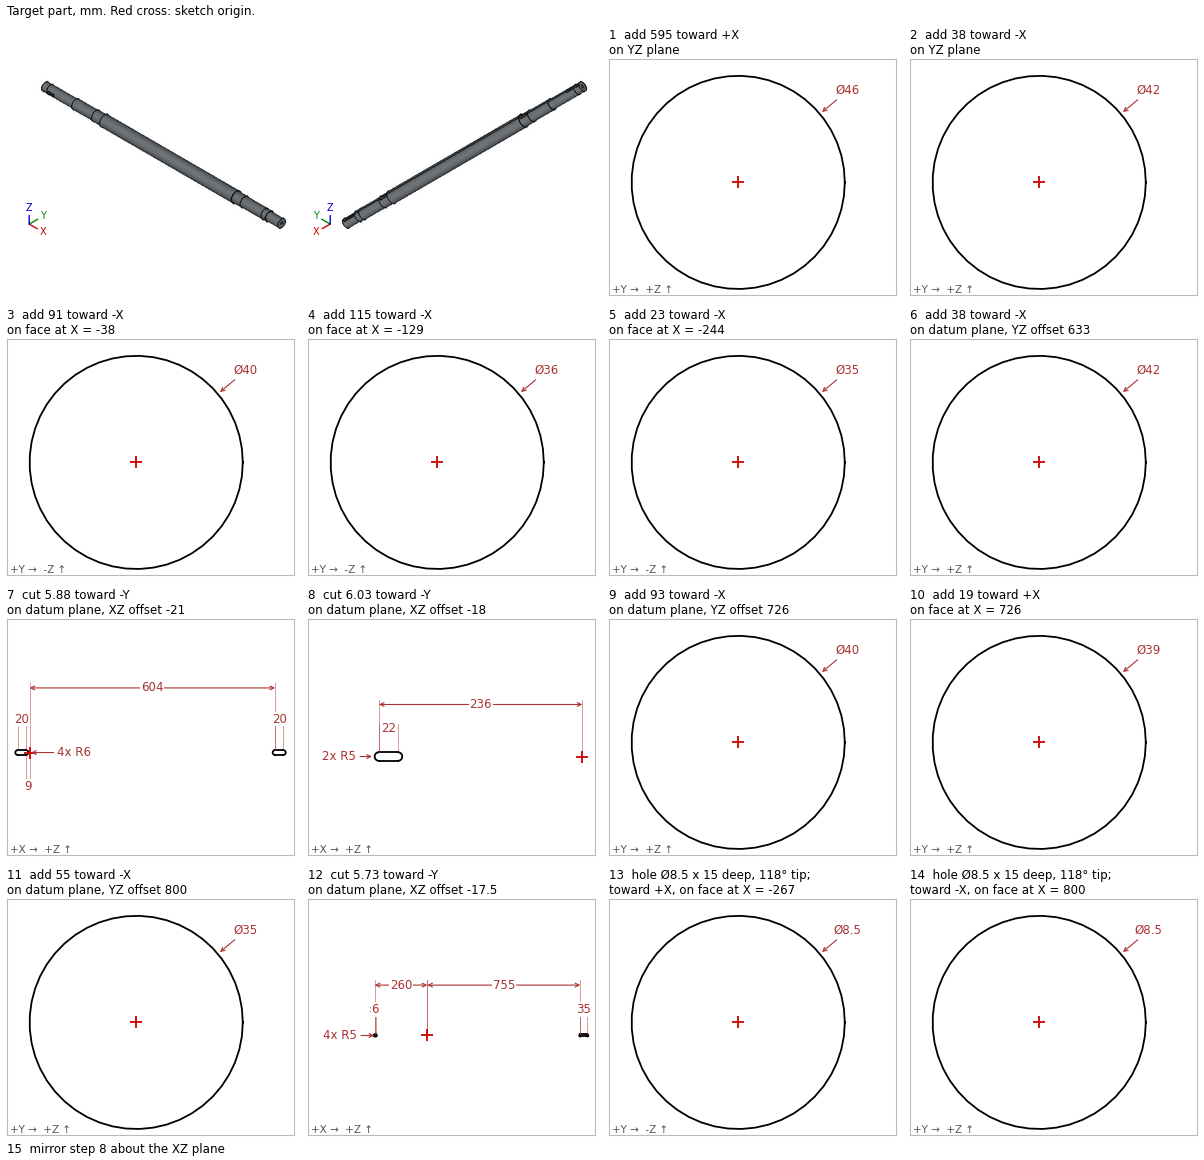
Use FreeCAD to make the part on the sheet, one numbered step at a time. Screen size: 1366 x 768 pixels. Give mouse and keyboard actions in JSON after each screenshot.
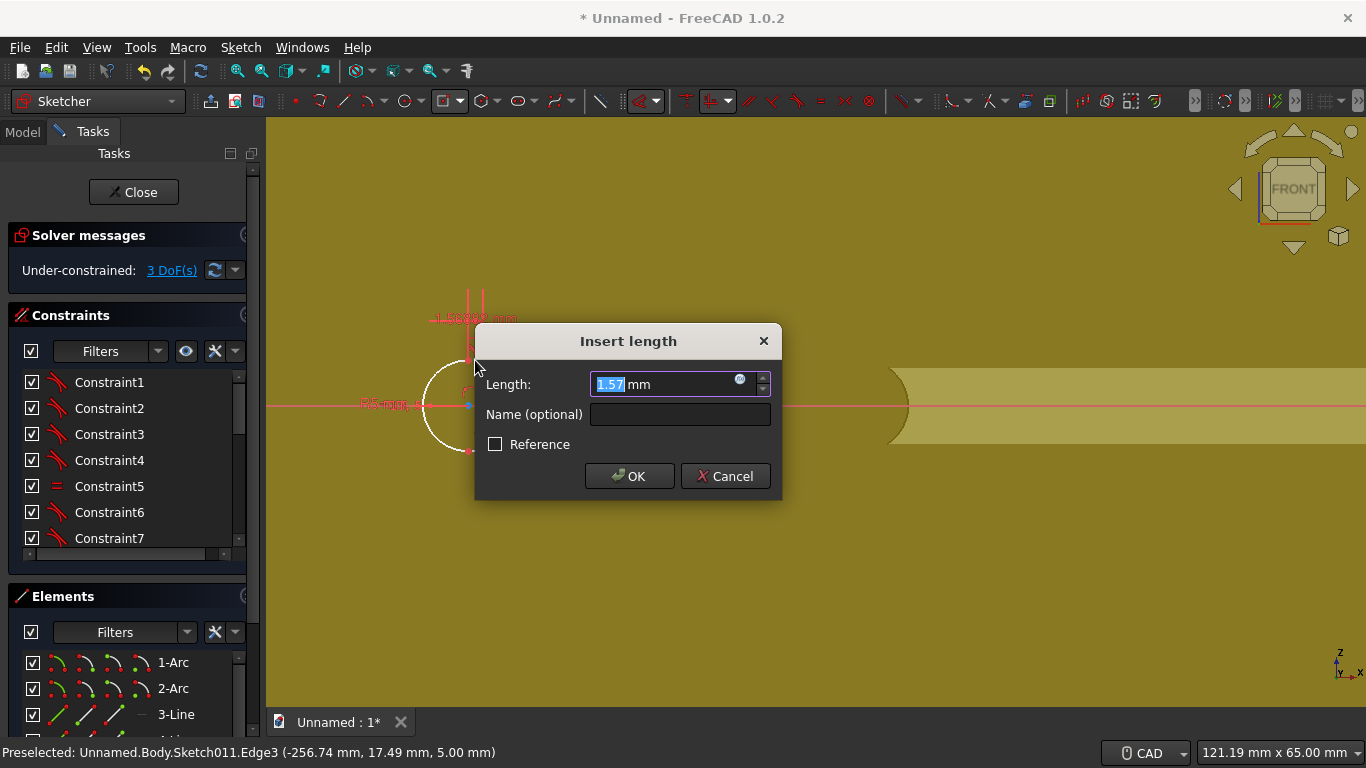
{"action": "type", "text": "6"}
{"action": "key", "text": "Return"}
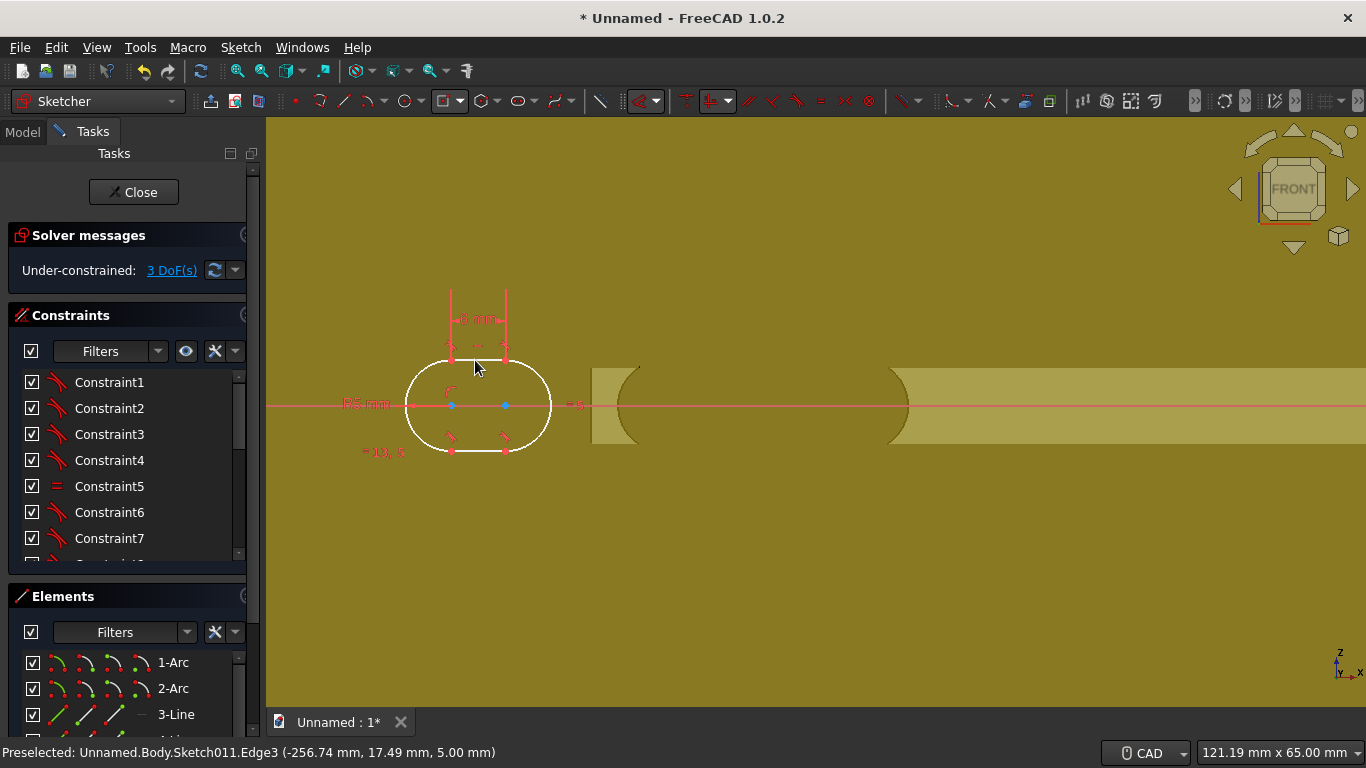
{"action": "scroll", "coordinate": [459, 412], "scroll_direction": "down", "scroll_amount": 14}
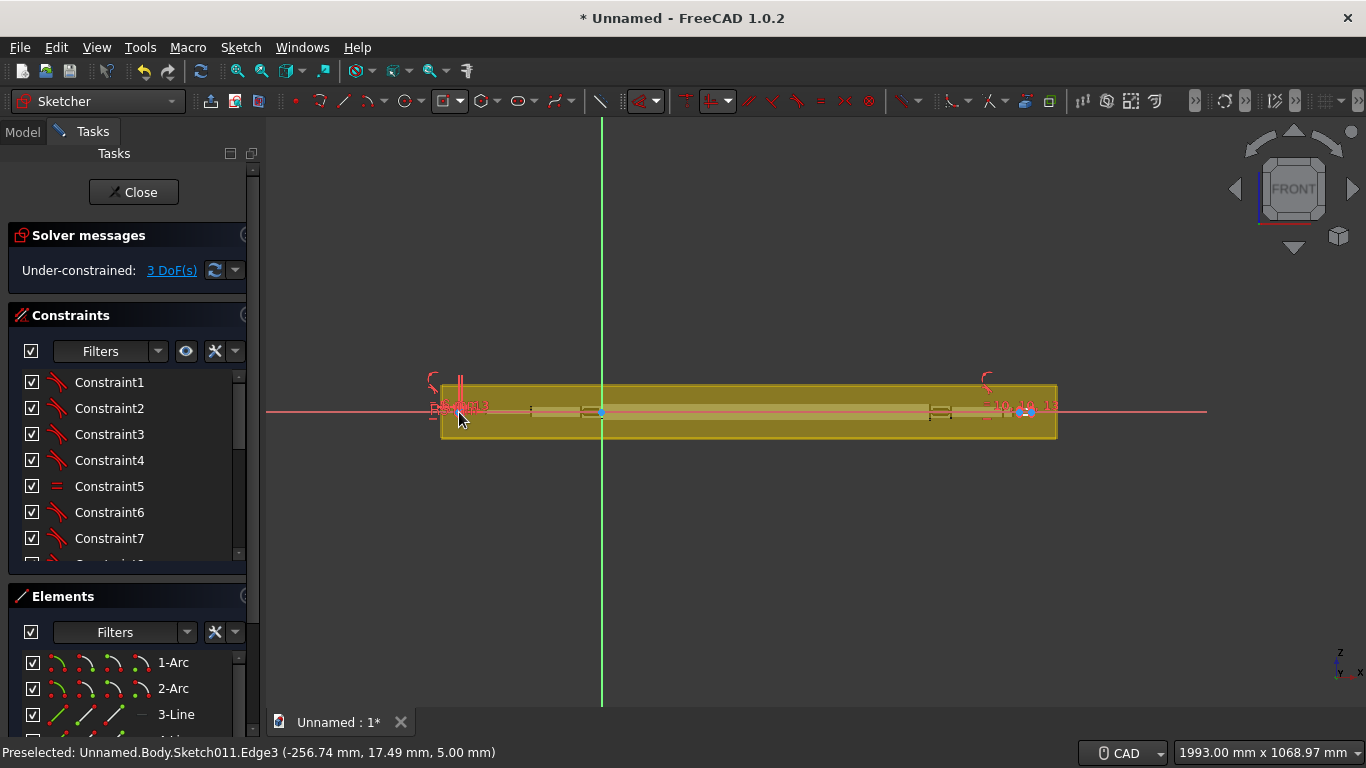
{"action": "scroll", "coordinate": [1023, 409], "scroll_direction": "up", "scroll_amount": 9}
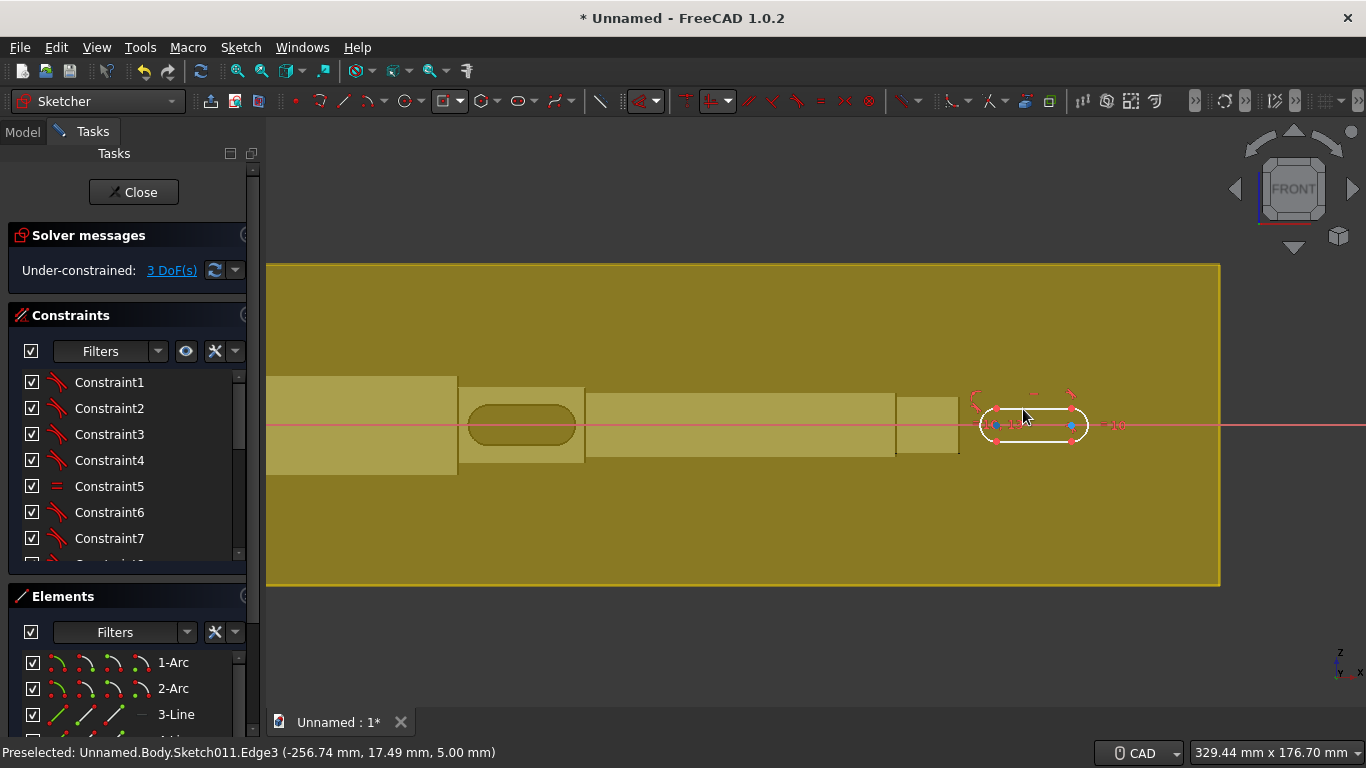
{"action": "left_click", "coordinate": [1049, 409]}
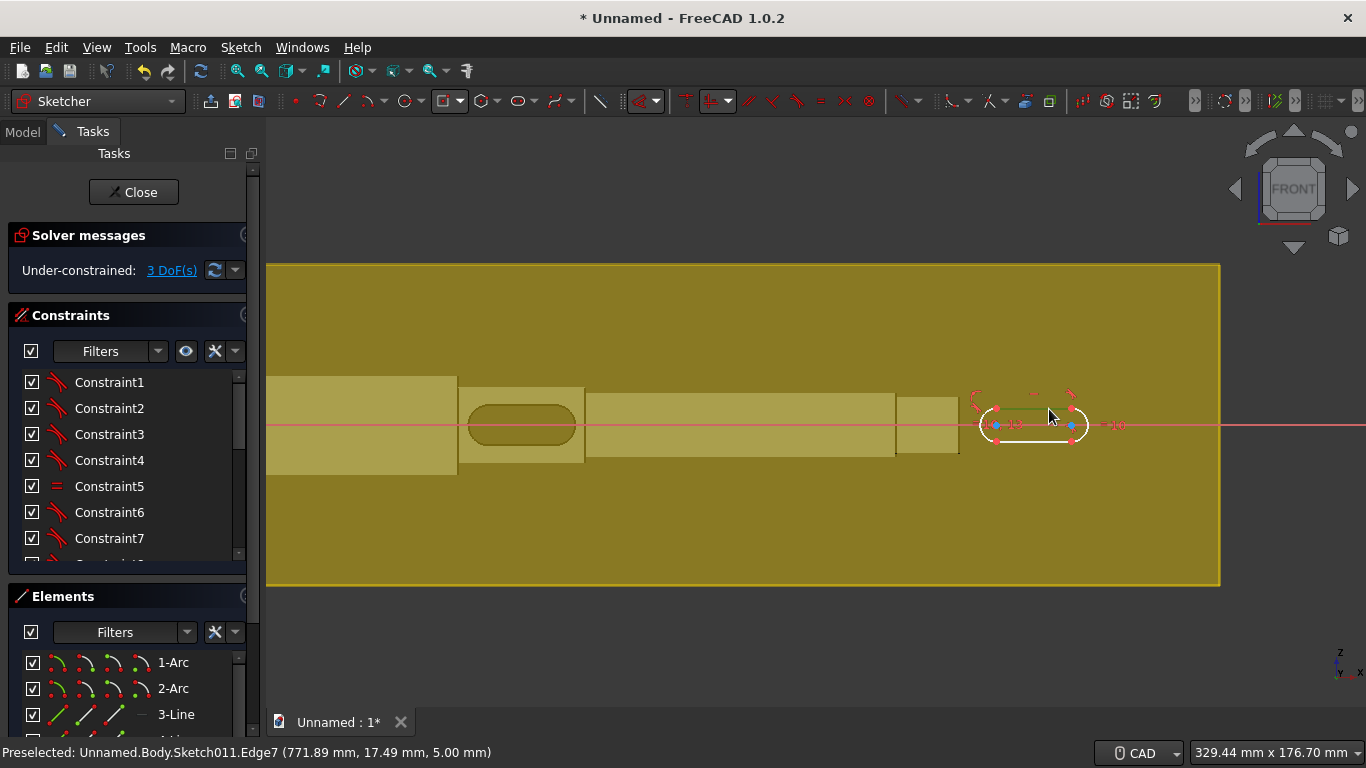
{"action": "key", "text": "l"}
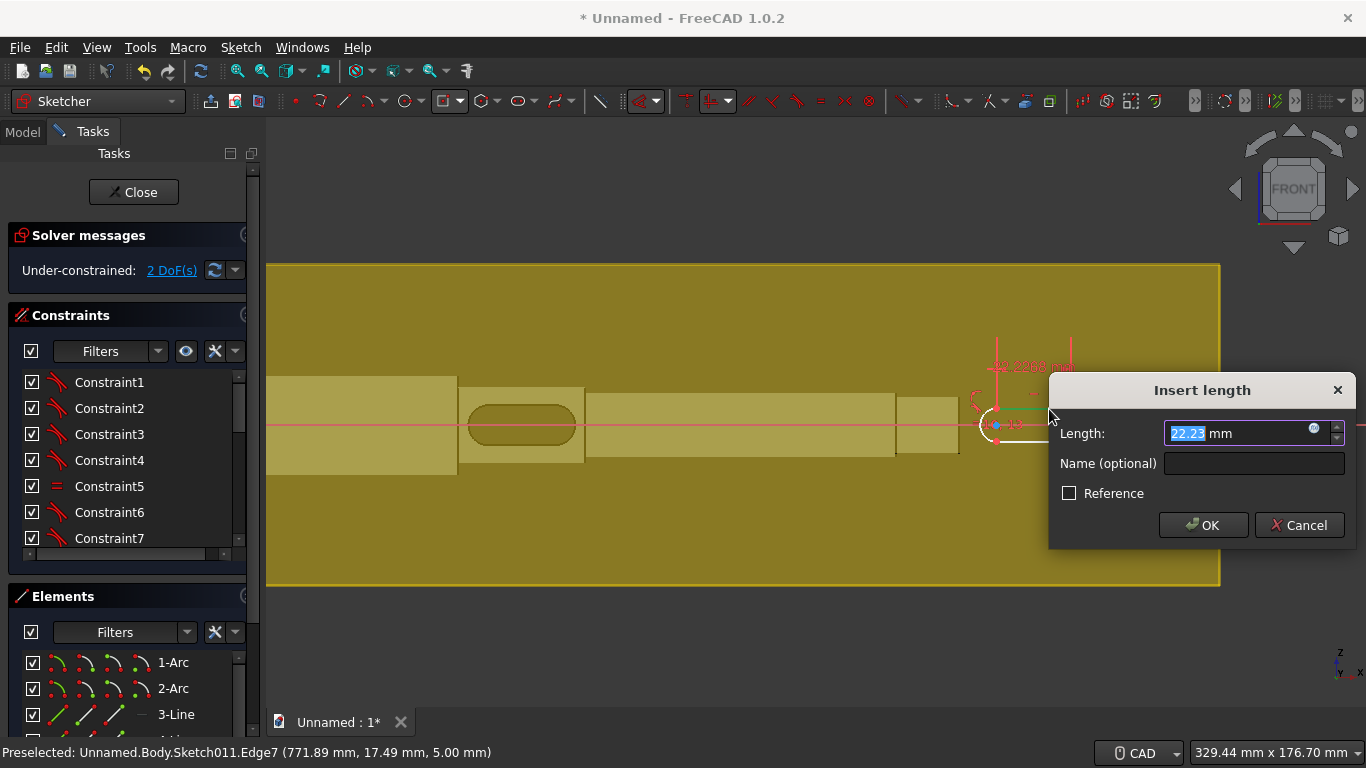
{"action": "type", "text": "35"}
{"action": "key", "text": "Return"}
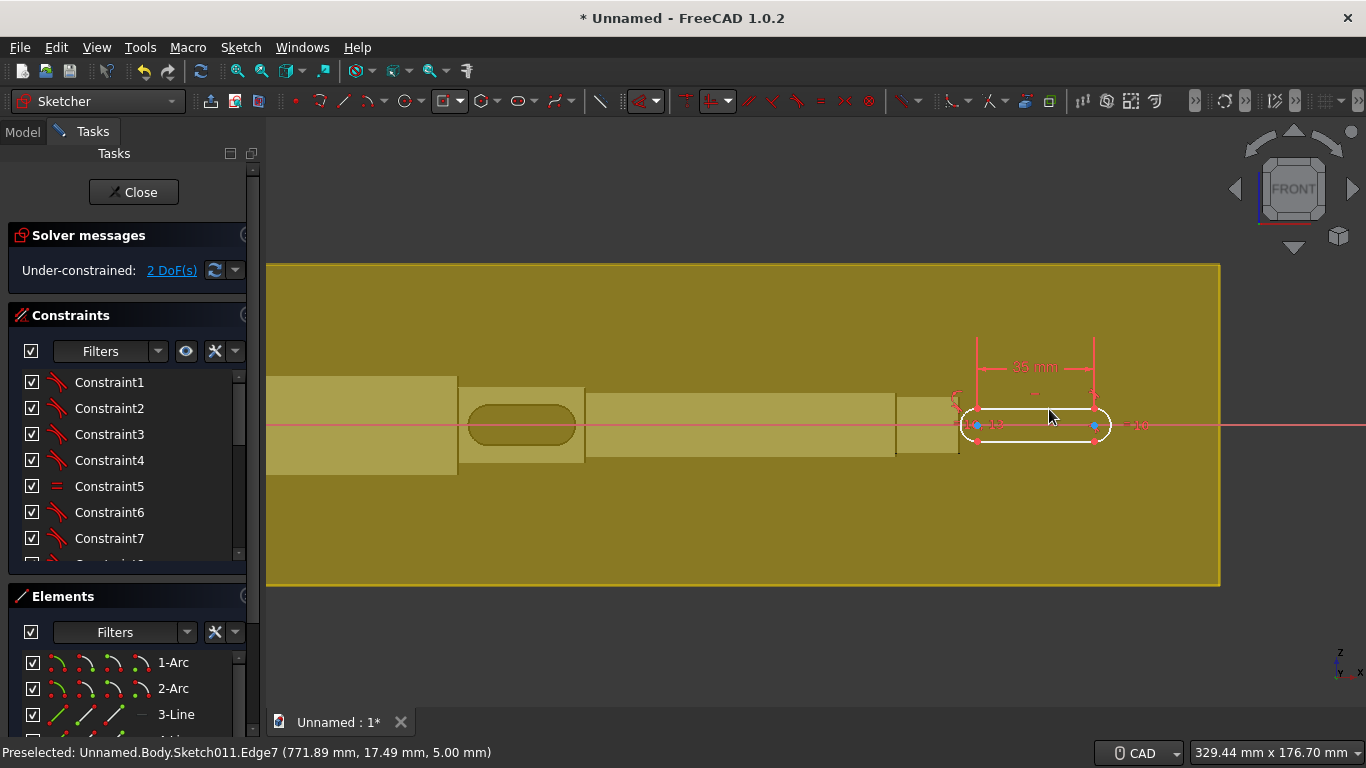
{"action": "scroll", "coordinate": [1023, 409], "scroll_direction": "down", "scroll_amount": 9}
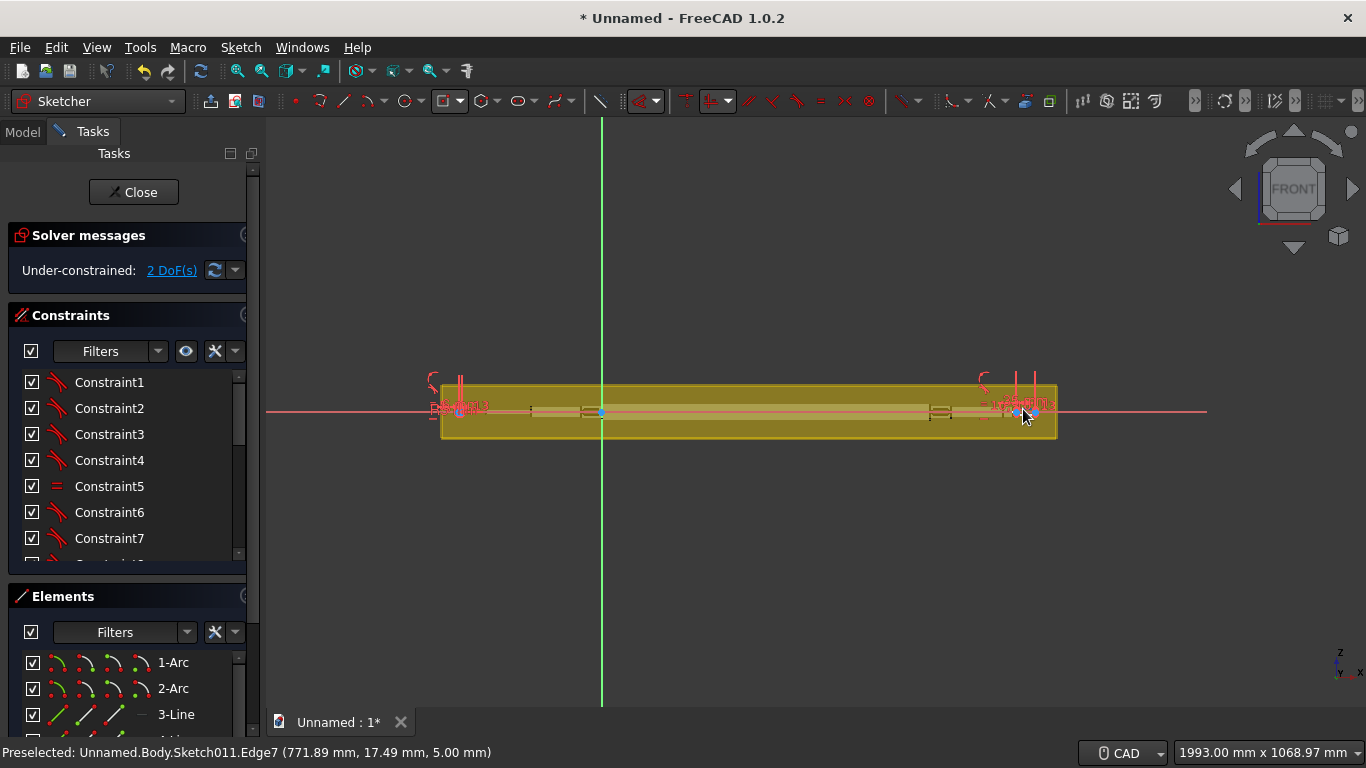
{"action": "scroll", "coordinate": [459, 409], "scroll_direction": "up", "scroll_amount": 8}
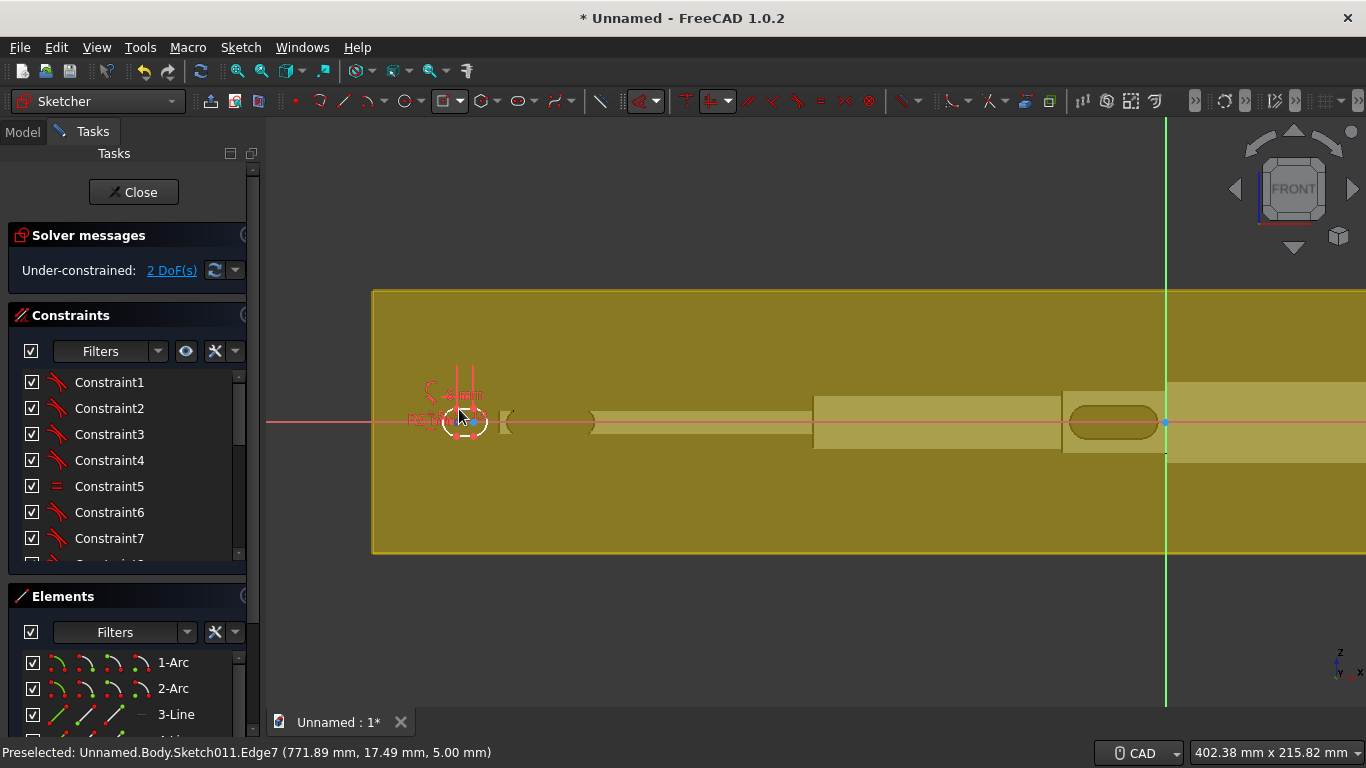
{"action": "left_click", "coordinate": [457, 409]}